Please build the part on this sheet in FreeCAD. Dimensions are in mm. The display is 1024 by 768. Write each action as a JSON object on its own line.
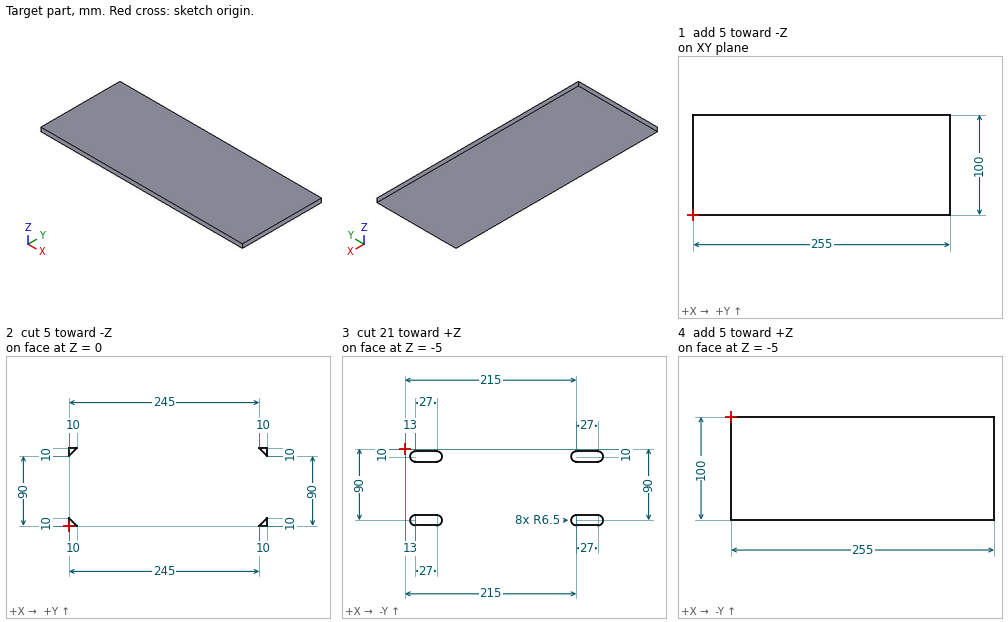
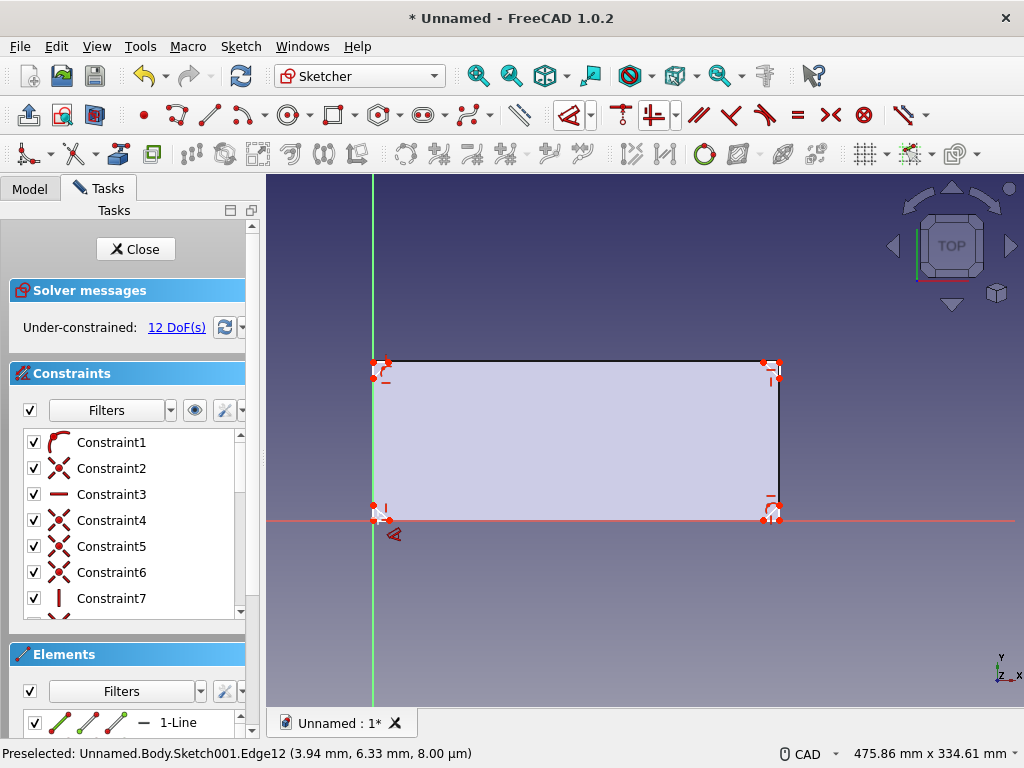
{"action": "scroll", "coordinate": [384, 362], "scroll_direction": "up", "scroll_amount": 8}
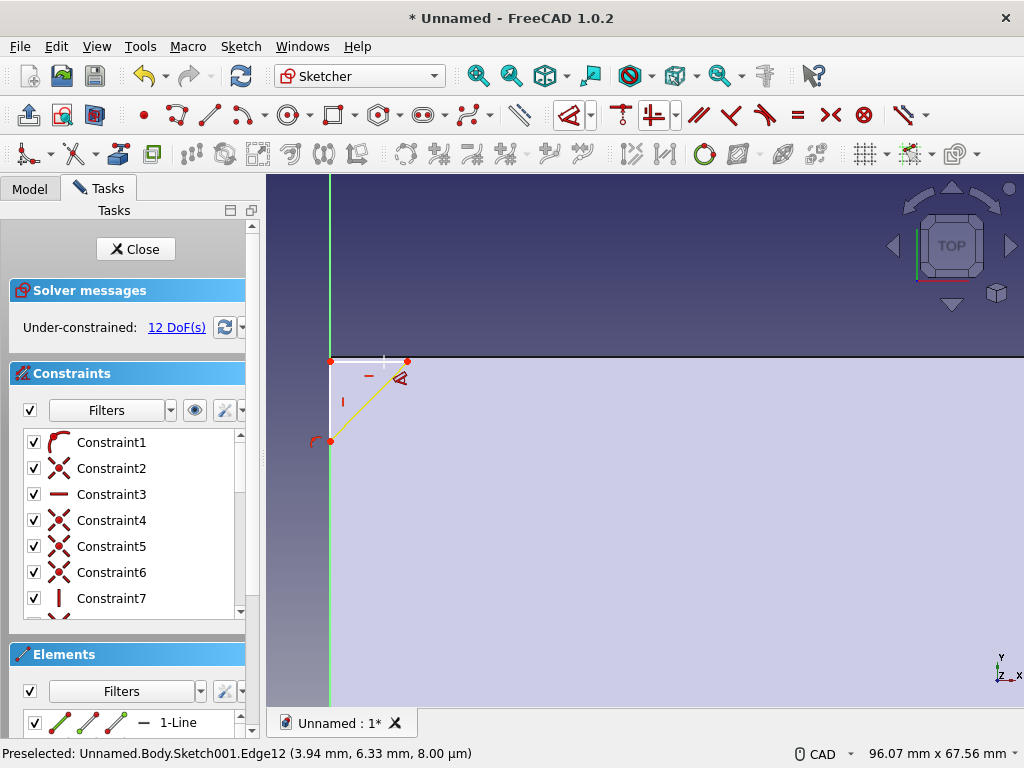
{"action": "left_click", "coordinate": [385, 362]}
{"action": "left_click", "coordinate": [369, 328]}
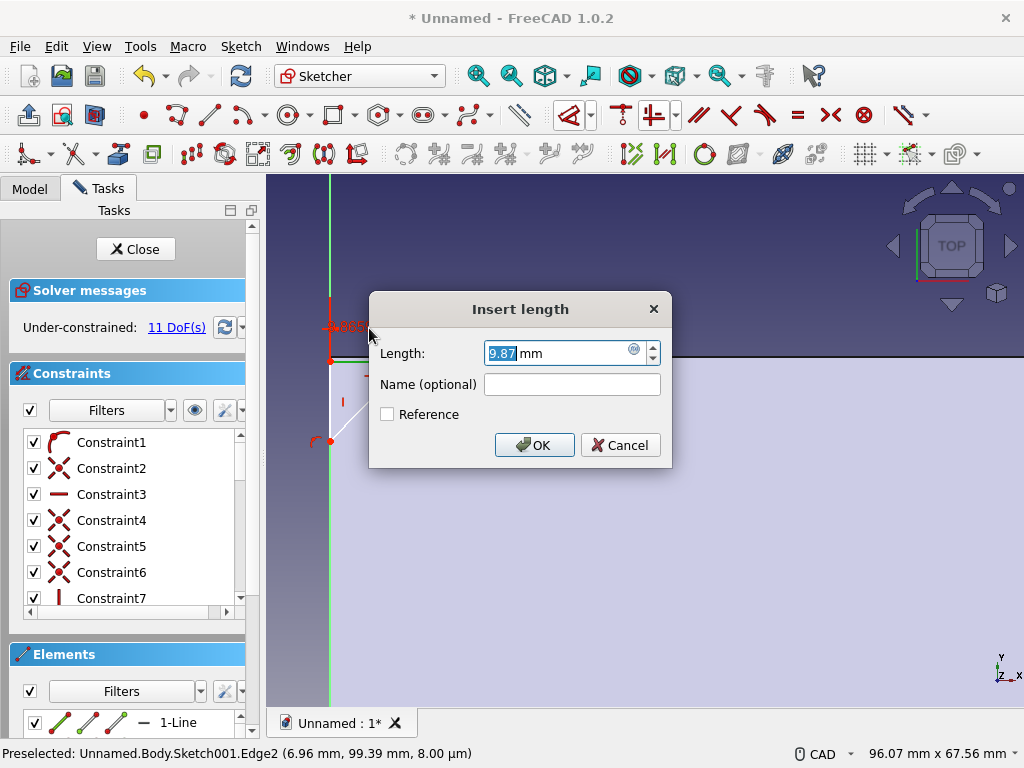
{"action": "type", "text": "10"}
{"action": "key", "text": "Return"}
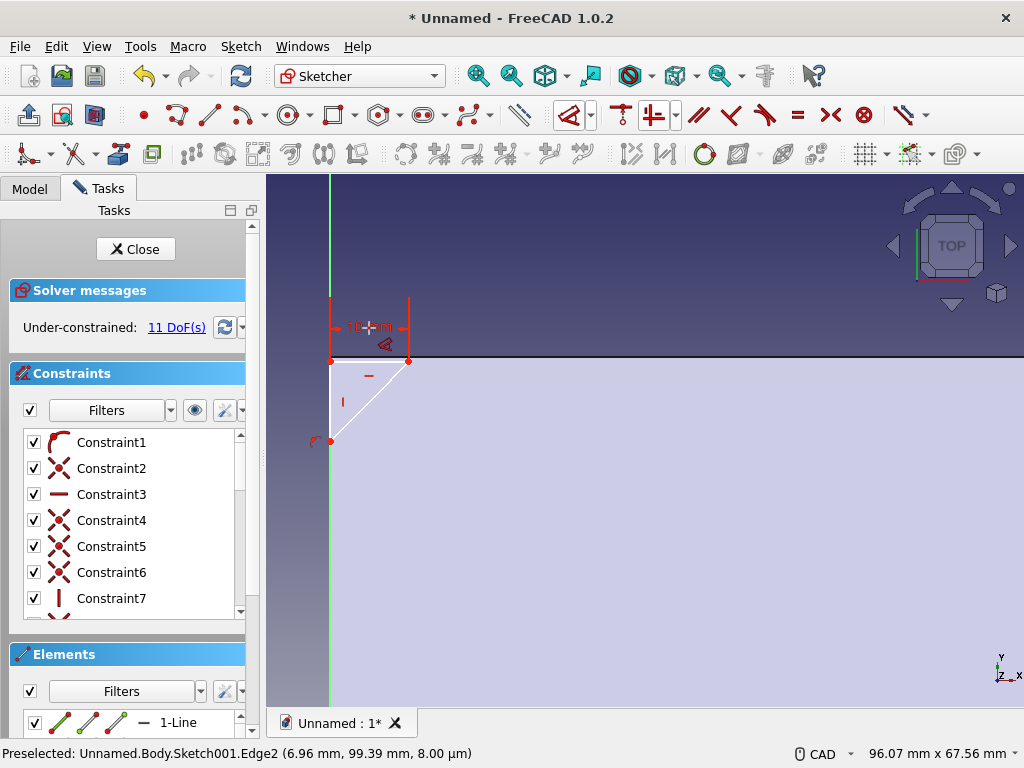
{"action": "left_click", "coordinate": [330, 386]}
{"action": "left_click", "coordinate": [296, 402]}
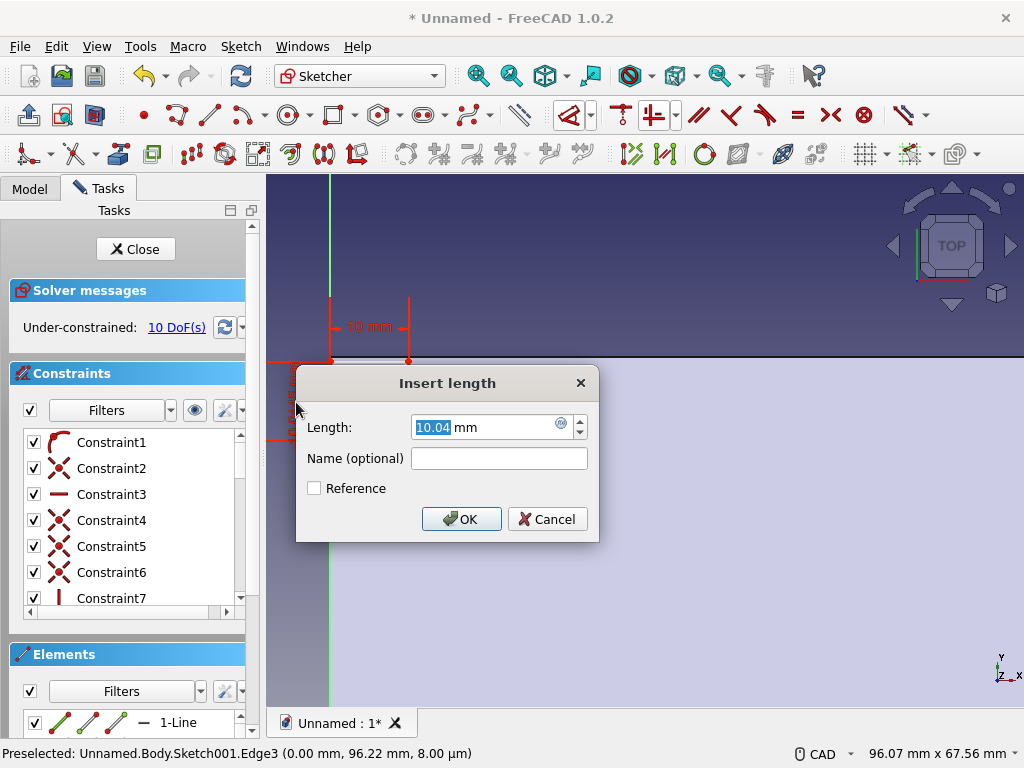
{"action": "type", "text": "10"}
{"action": "key", "text": "Return"}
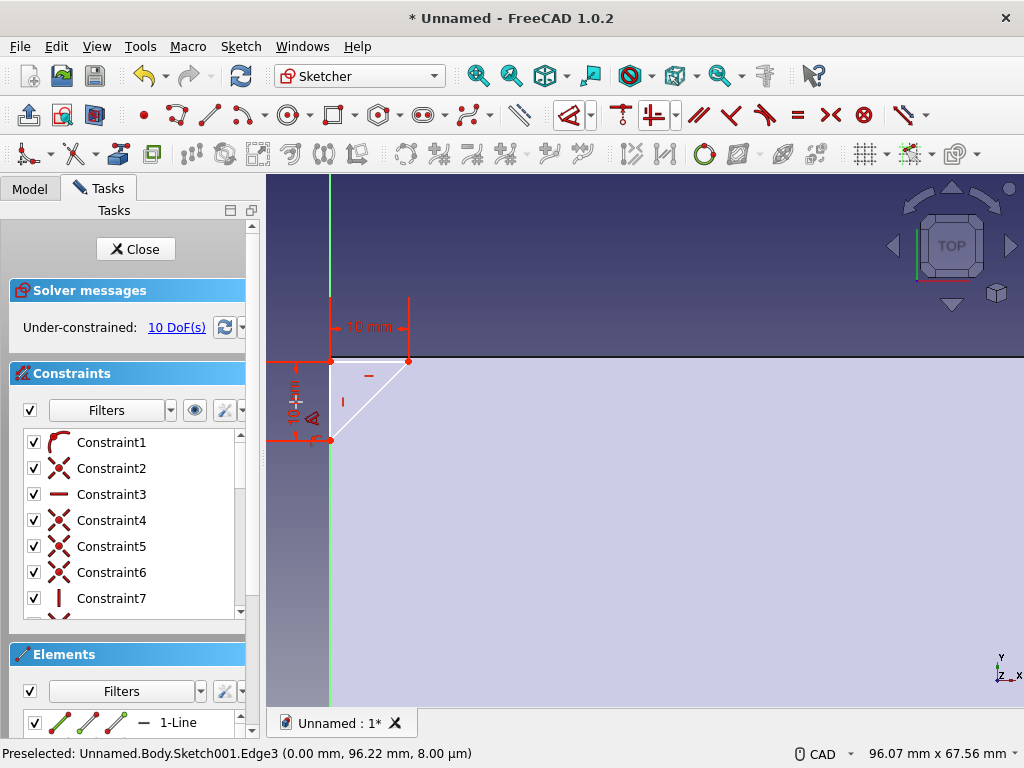
{"action": "scroll", "coordinate": [384, 362], "scroll_direction": "down", "scroll_amount": 8}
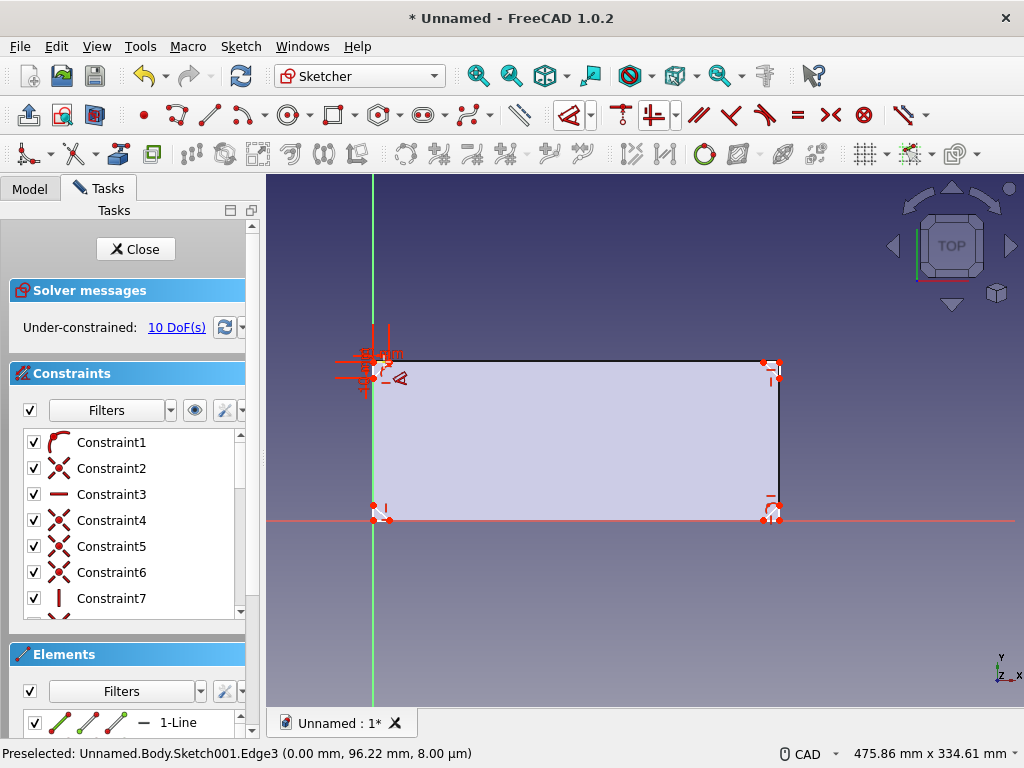
{"action": "scroll", "coordinate": [780, 373], "scroll_direction": "up", "scroll_amount": 7}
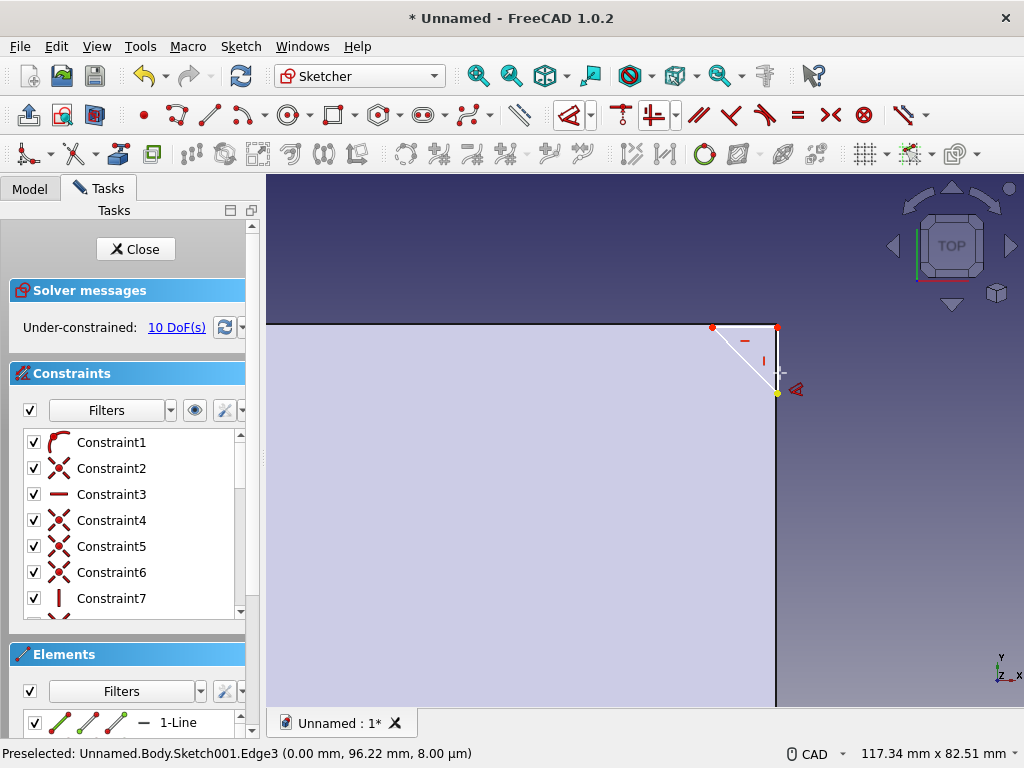
{"action": "left_click", "coordinate": [778, 373]}
{"action": "left_click", "coordinate": [812, 360]}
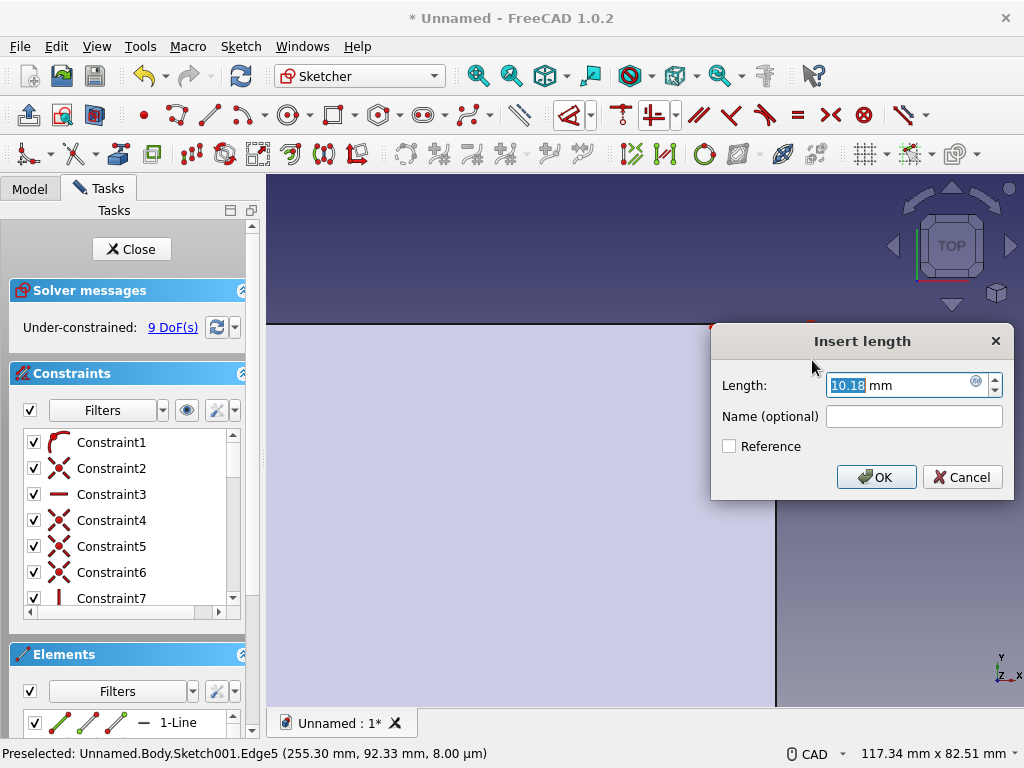
{"action": "type", "text": "10"}
{"action": "key", "text": "Return"}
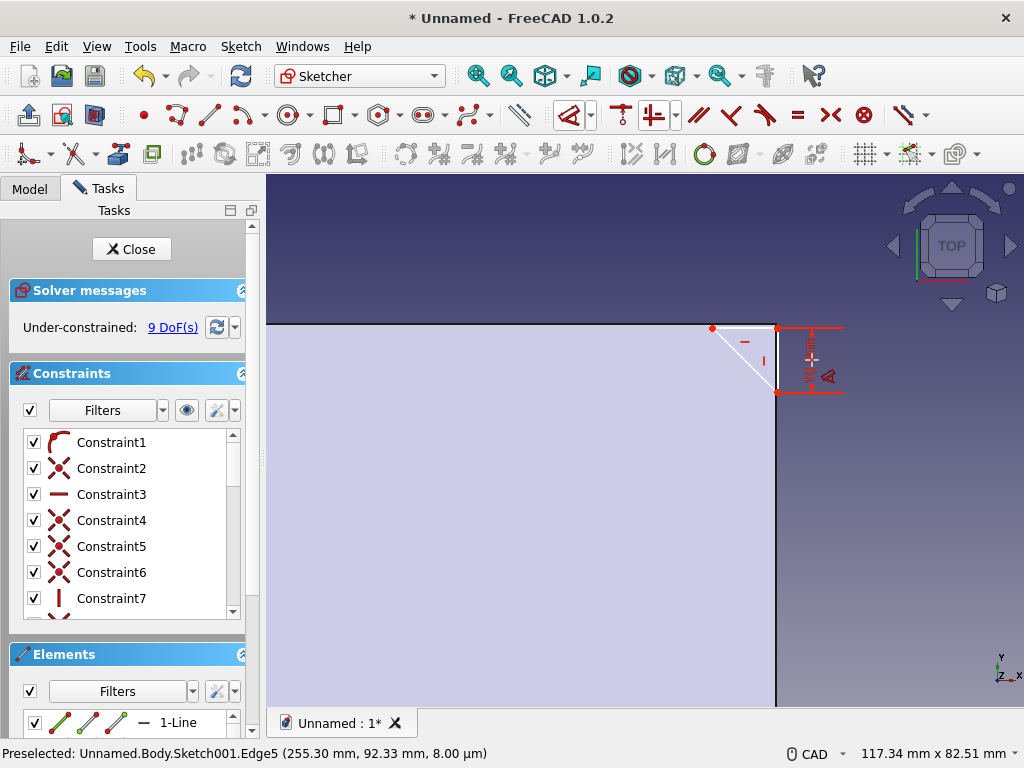
{"action": "left_click", "coordinate": [758, 328]}
{"action": "left_click", "coordinate": [745, 294]}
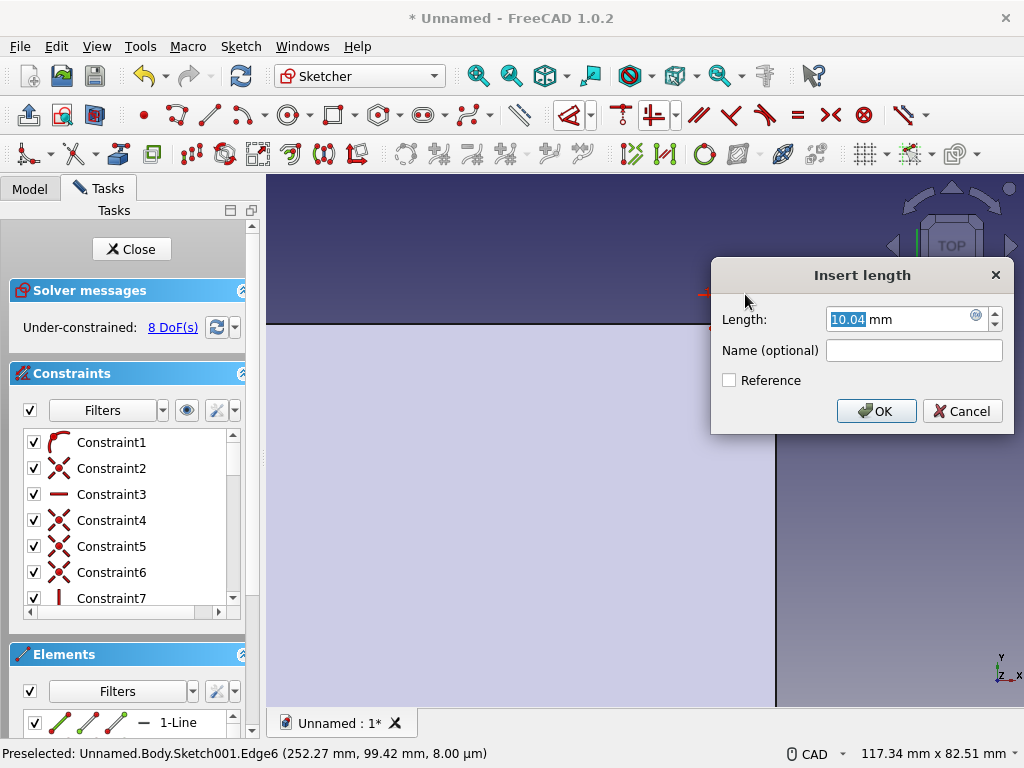
{"action": "type", "text": "10"}
{"action": "key", "text": "Return"}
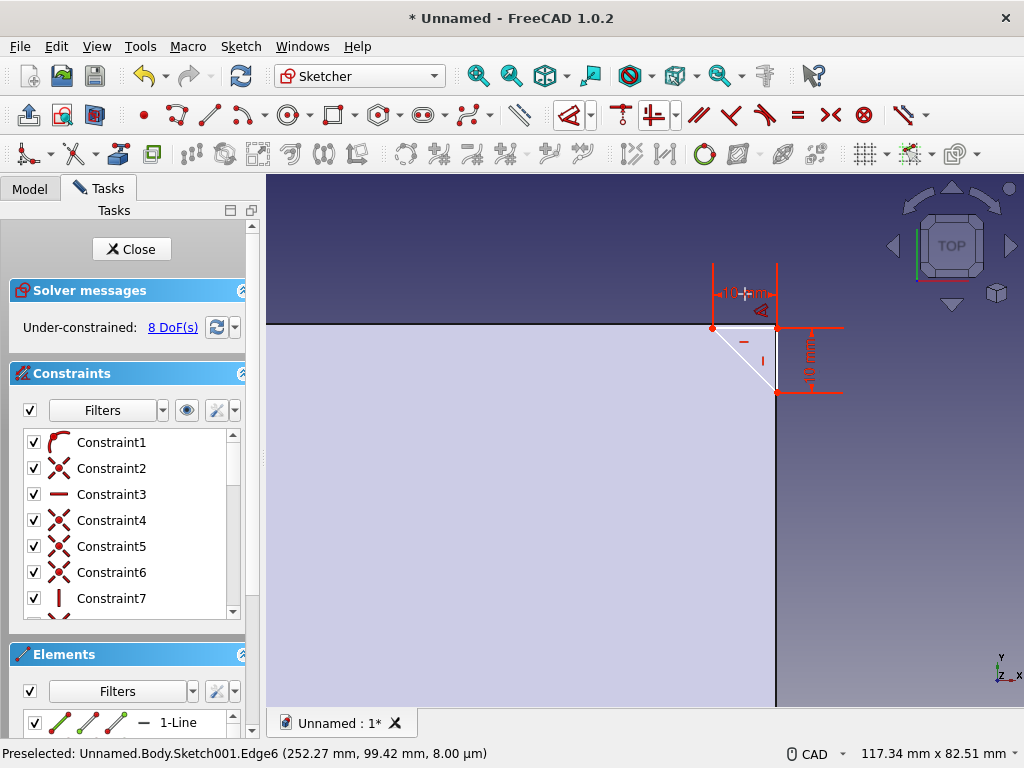
{"action": "scroll", "coordinate": [781, 373], "scroll_direction": "down", "scroll_amount": 7}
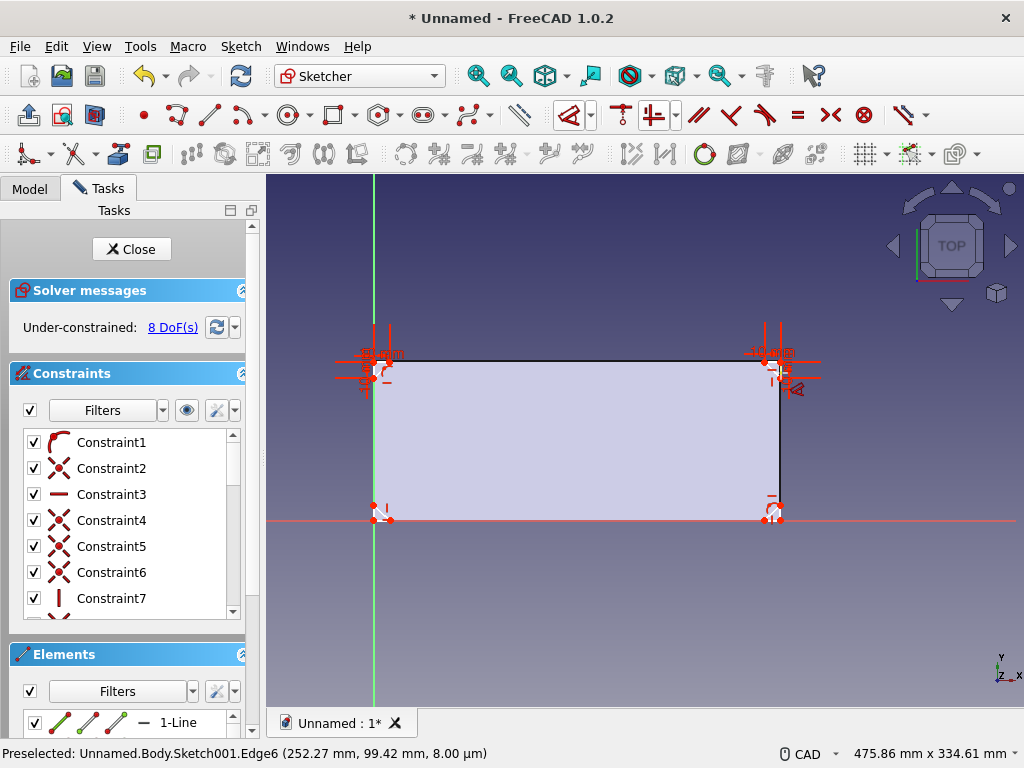
{"action": "scroll", "coordinate": [769, 521], "scroll_direction": "up", "scroll_amount": 8}